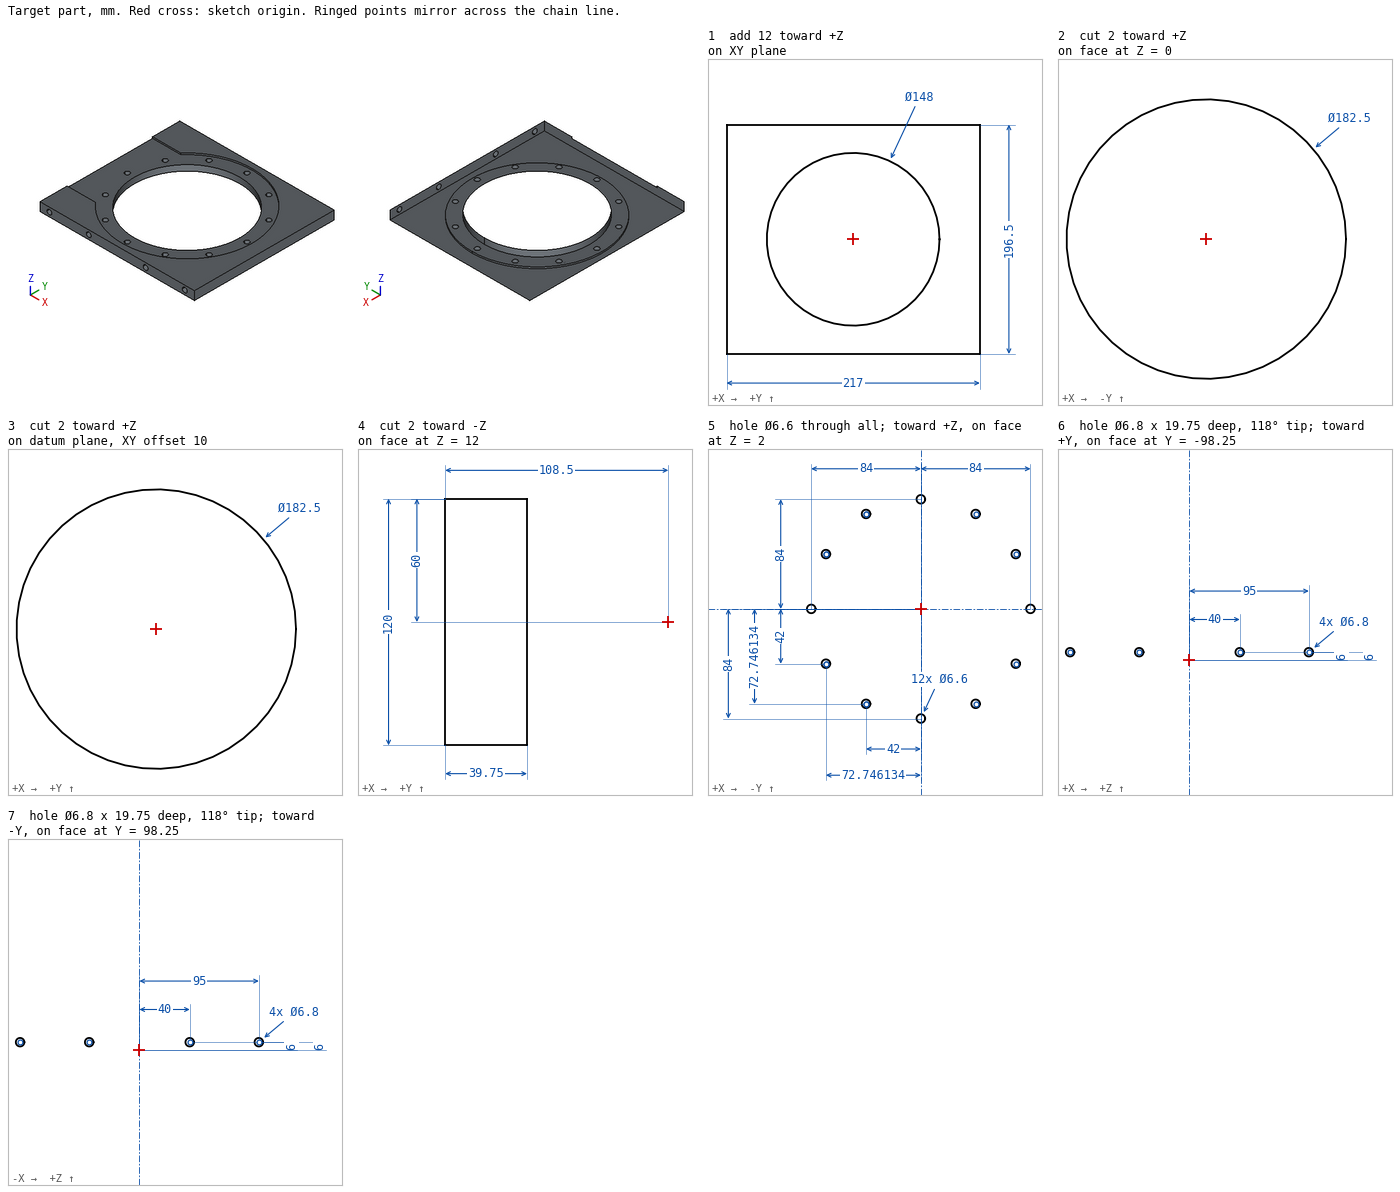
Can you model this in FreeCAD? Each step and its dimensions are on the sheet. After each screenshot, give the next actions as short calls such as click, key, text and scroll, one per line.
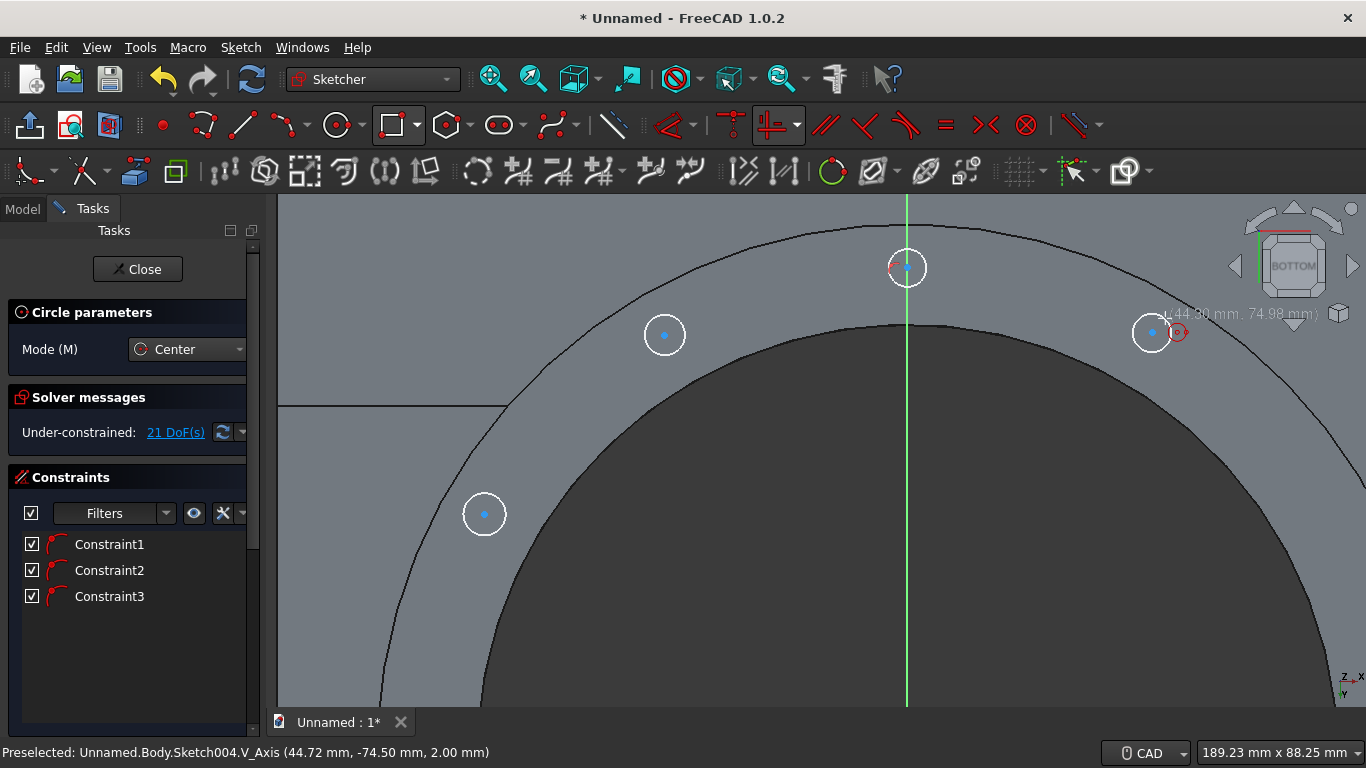
scroll(679, 319, down, 6)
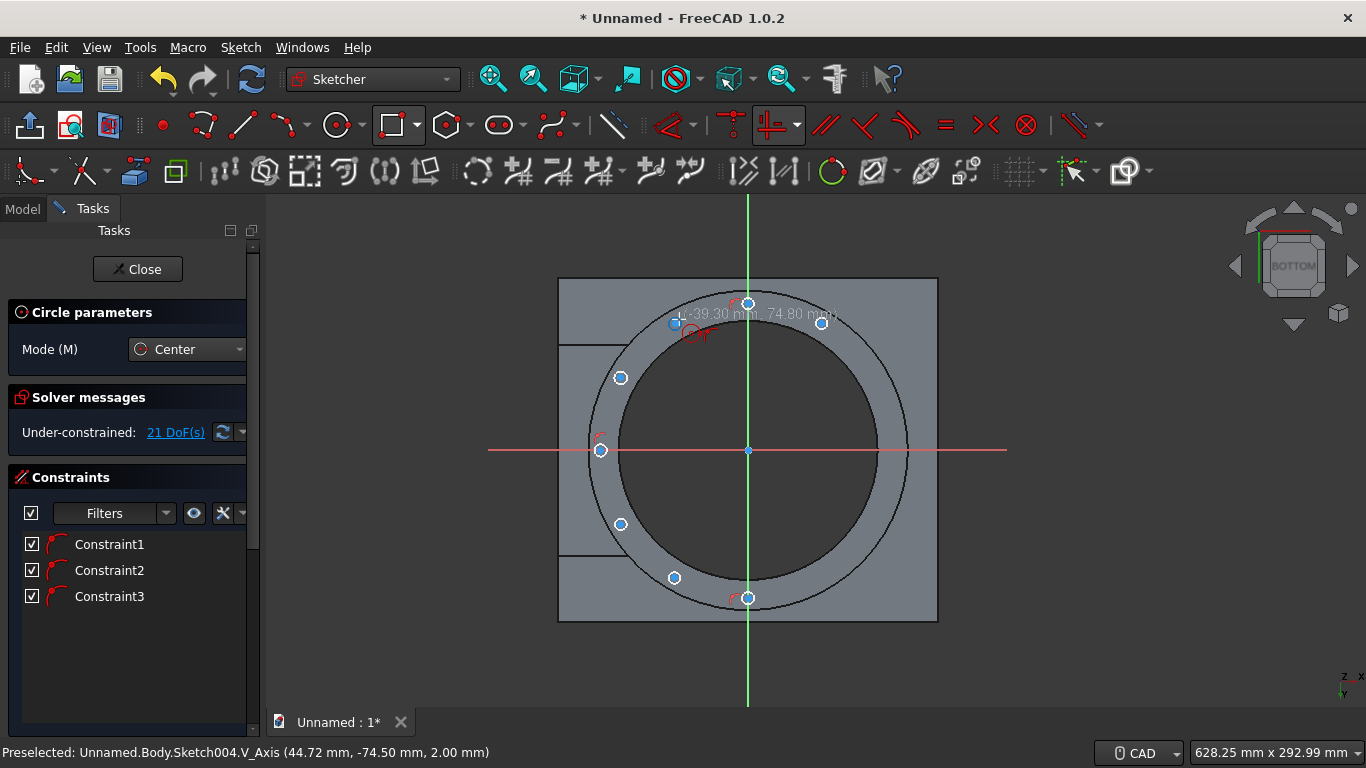
scroll(875, 377, up, 7)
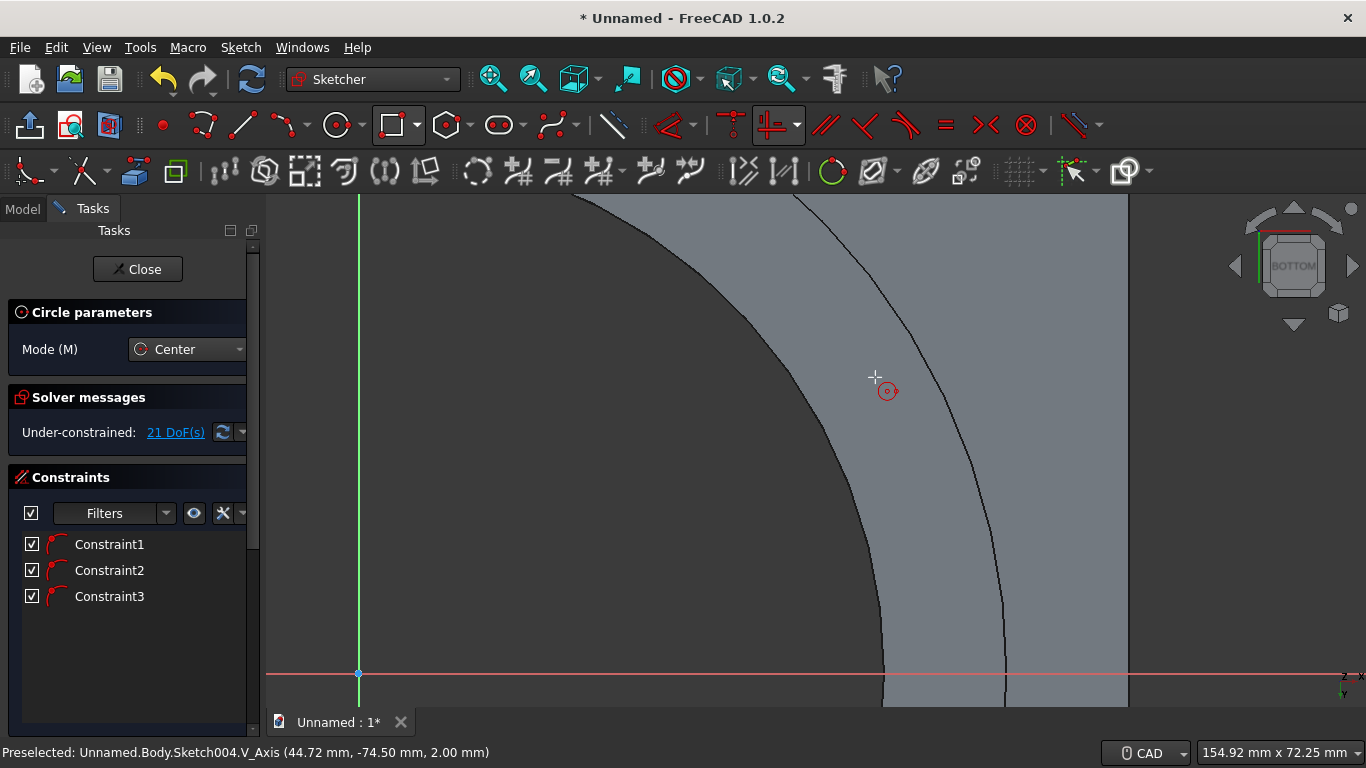
scroll(875, 377, down, 7)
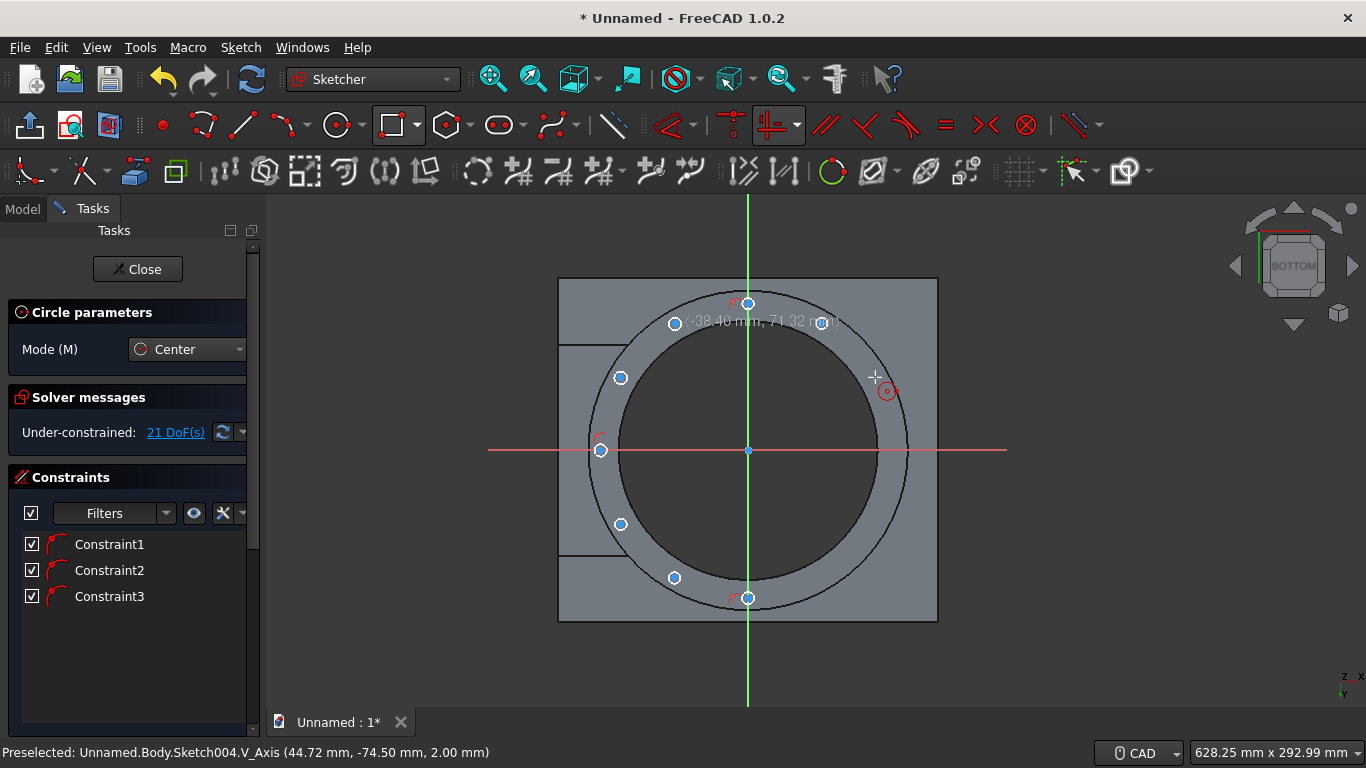
click(875, 377)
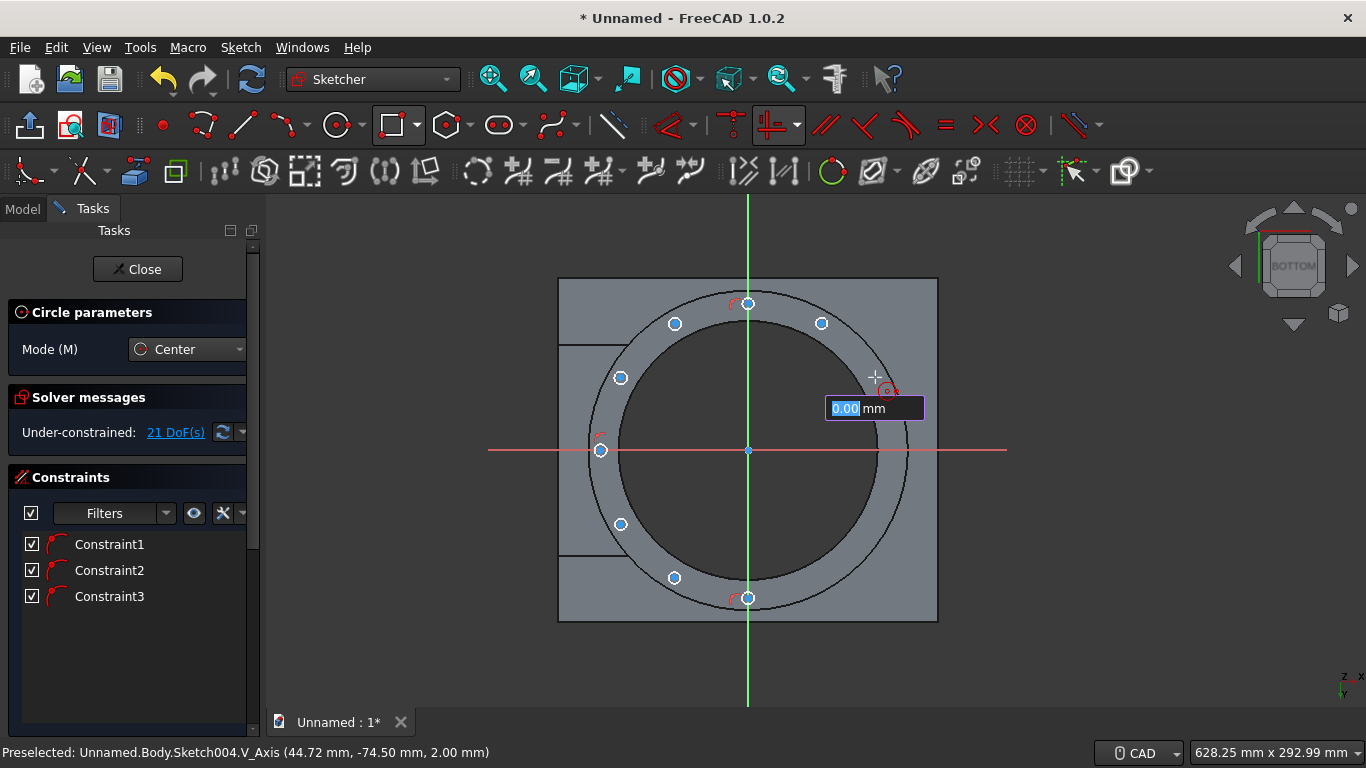
scroll(880, 373, up, 6)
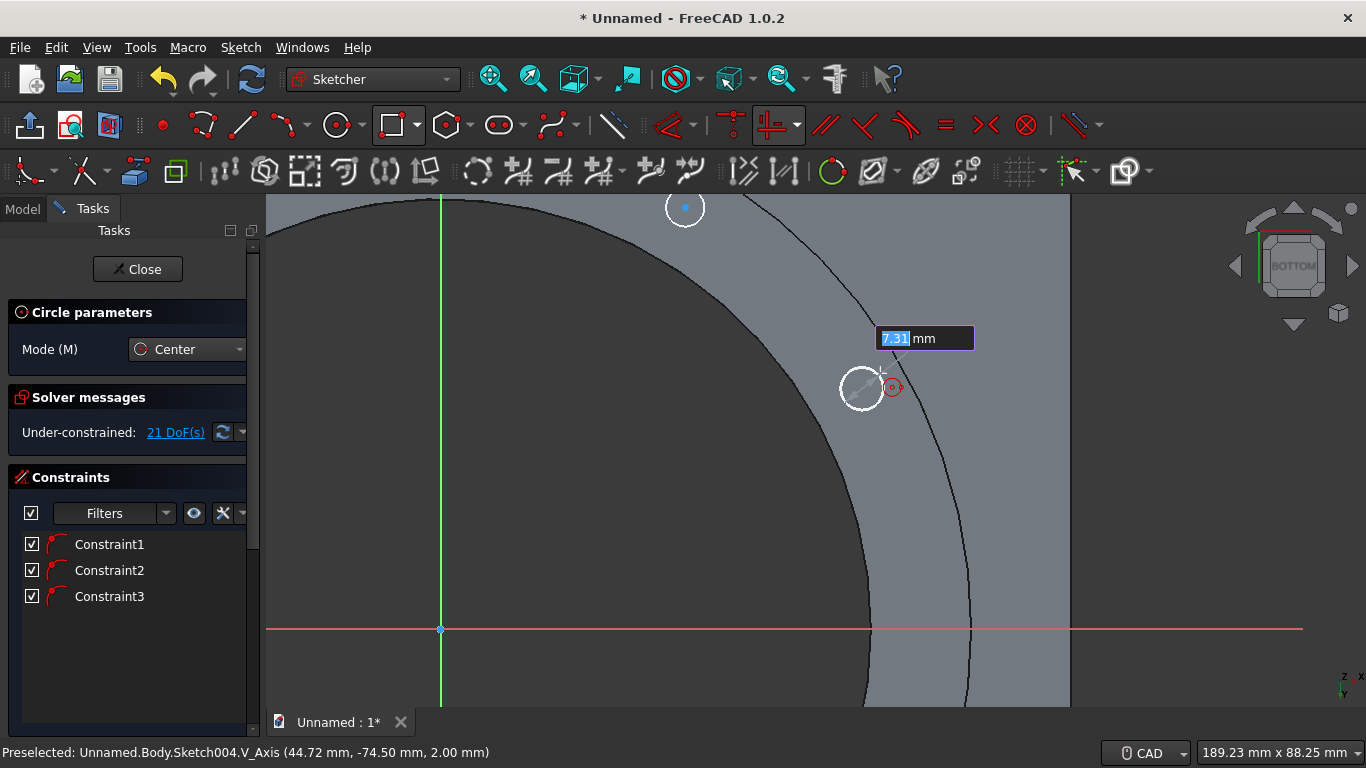
click(877, 372)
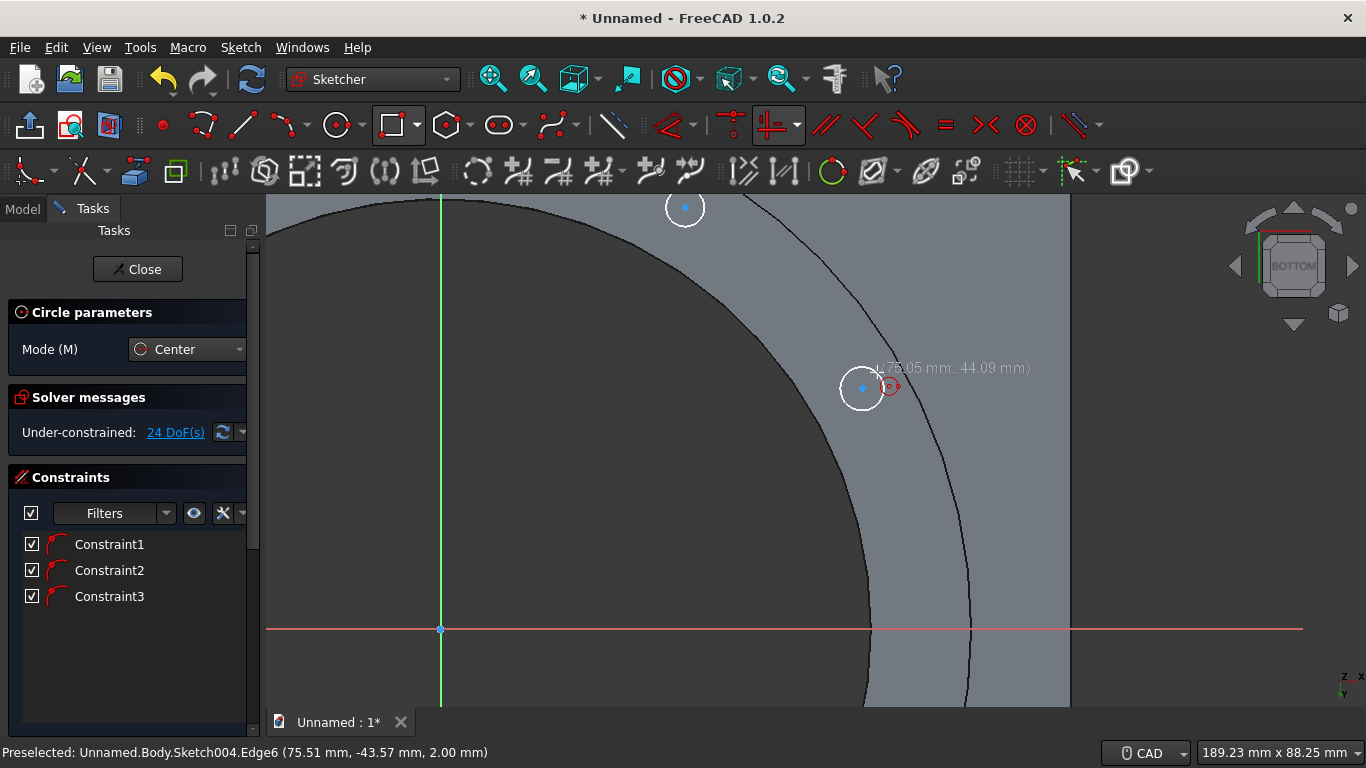
click(929, 629)
click(936, 611)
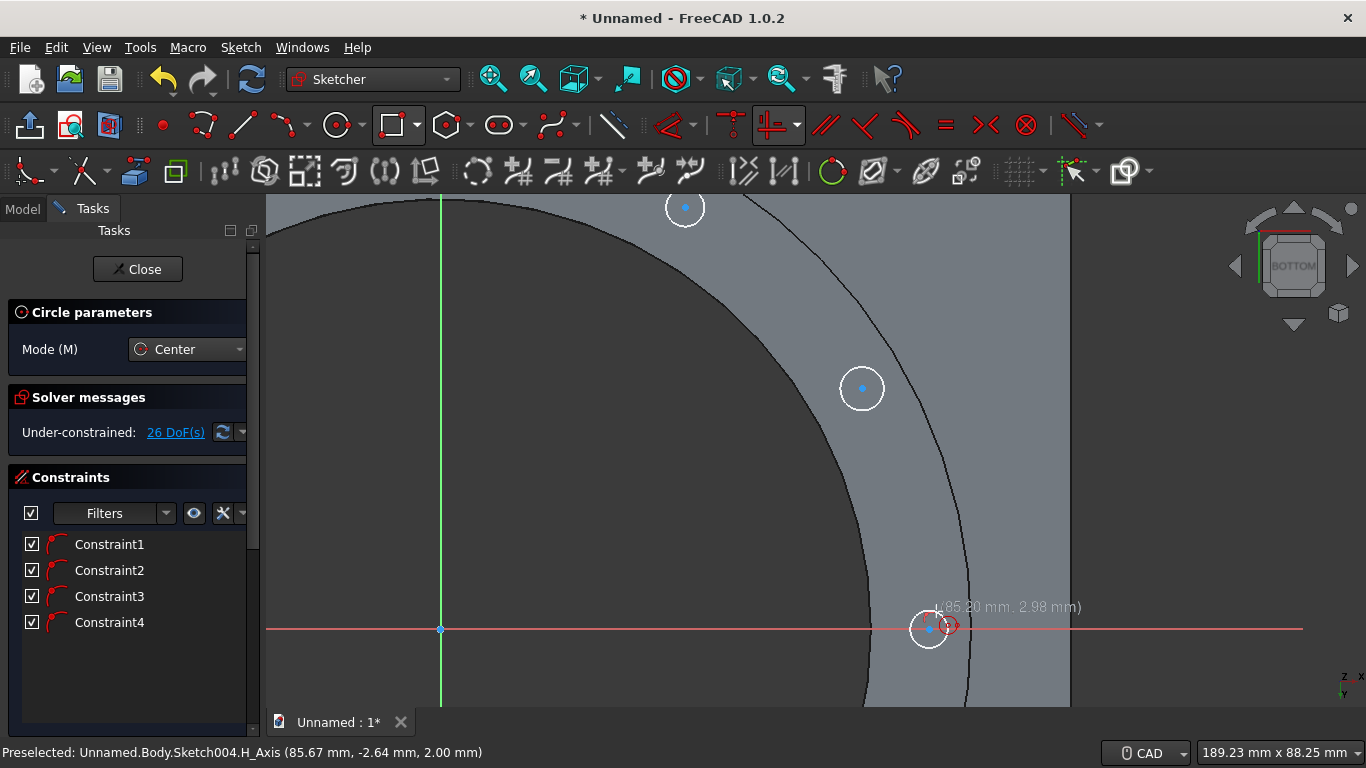
scroll(880, 373, down, 6)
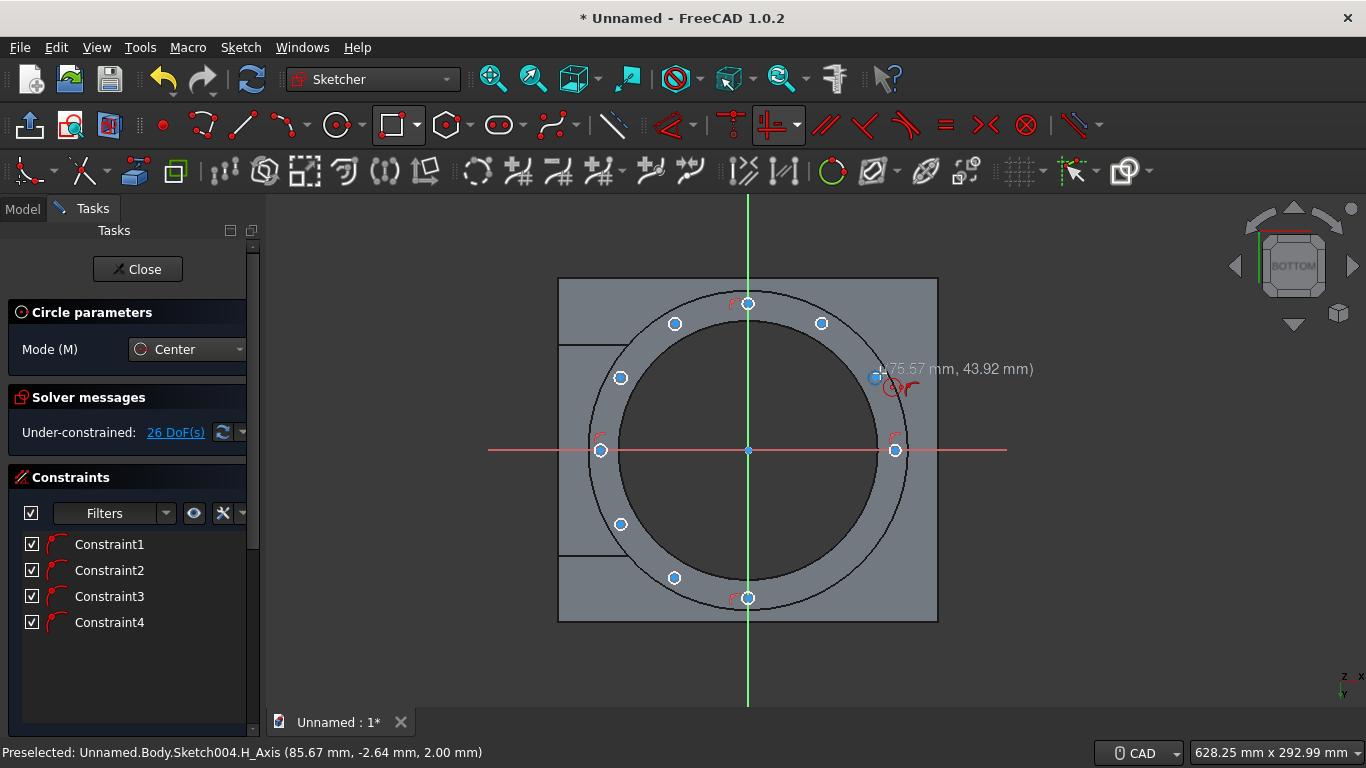
scroll(875, 524, up, 7)